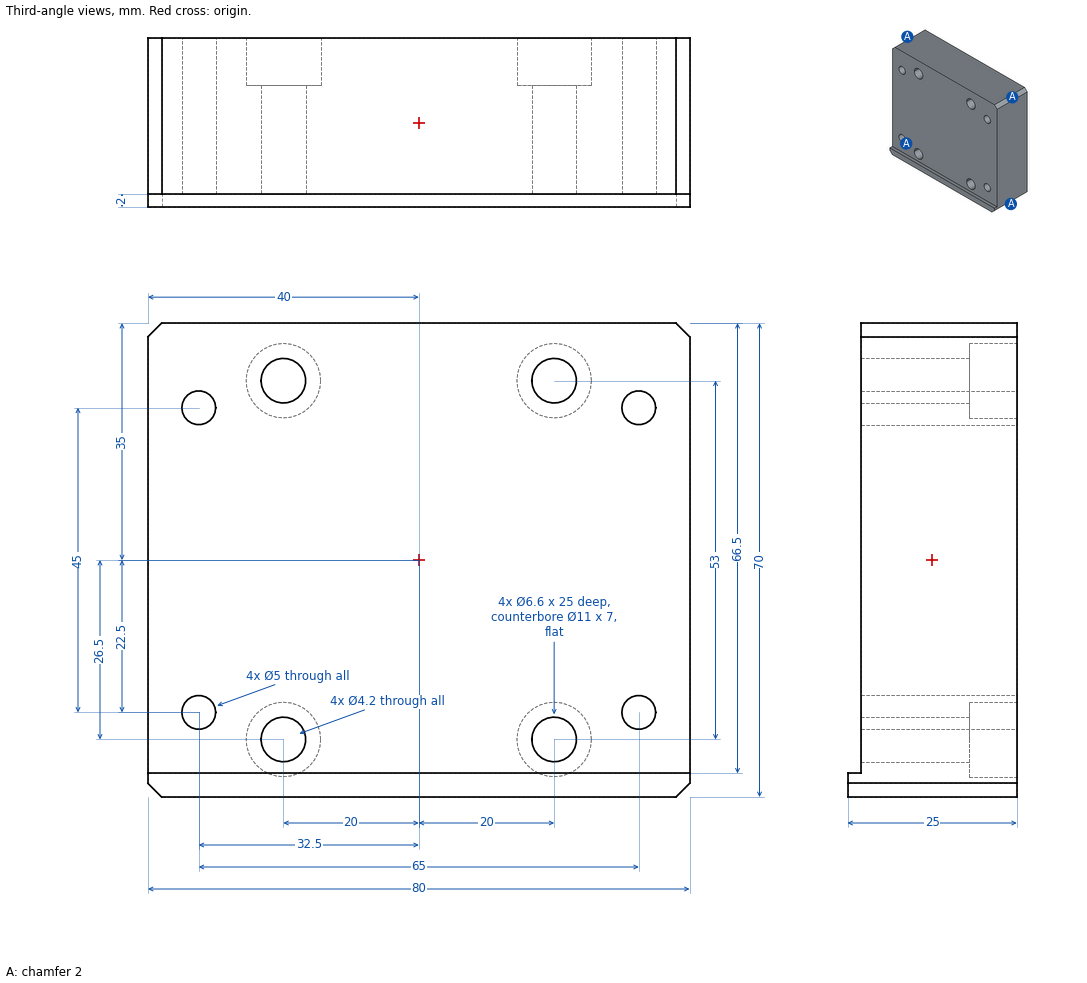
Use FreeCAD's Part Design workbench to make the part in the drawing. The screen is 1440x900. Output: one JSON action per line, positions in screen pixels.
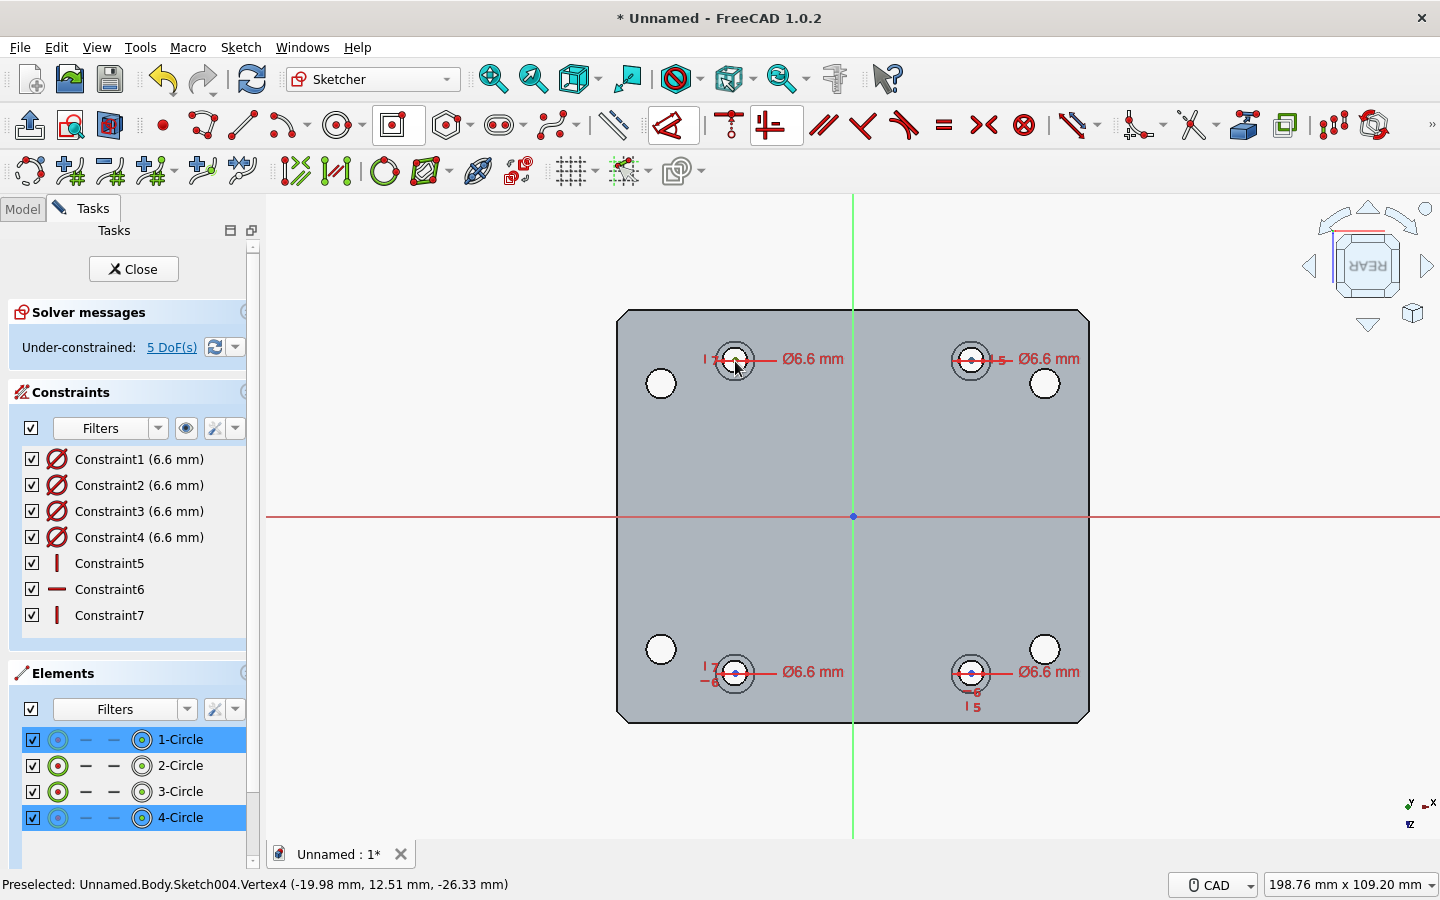
{"action": "key", "text": "h"}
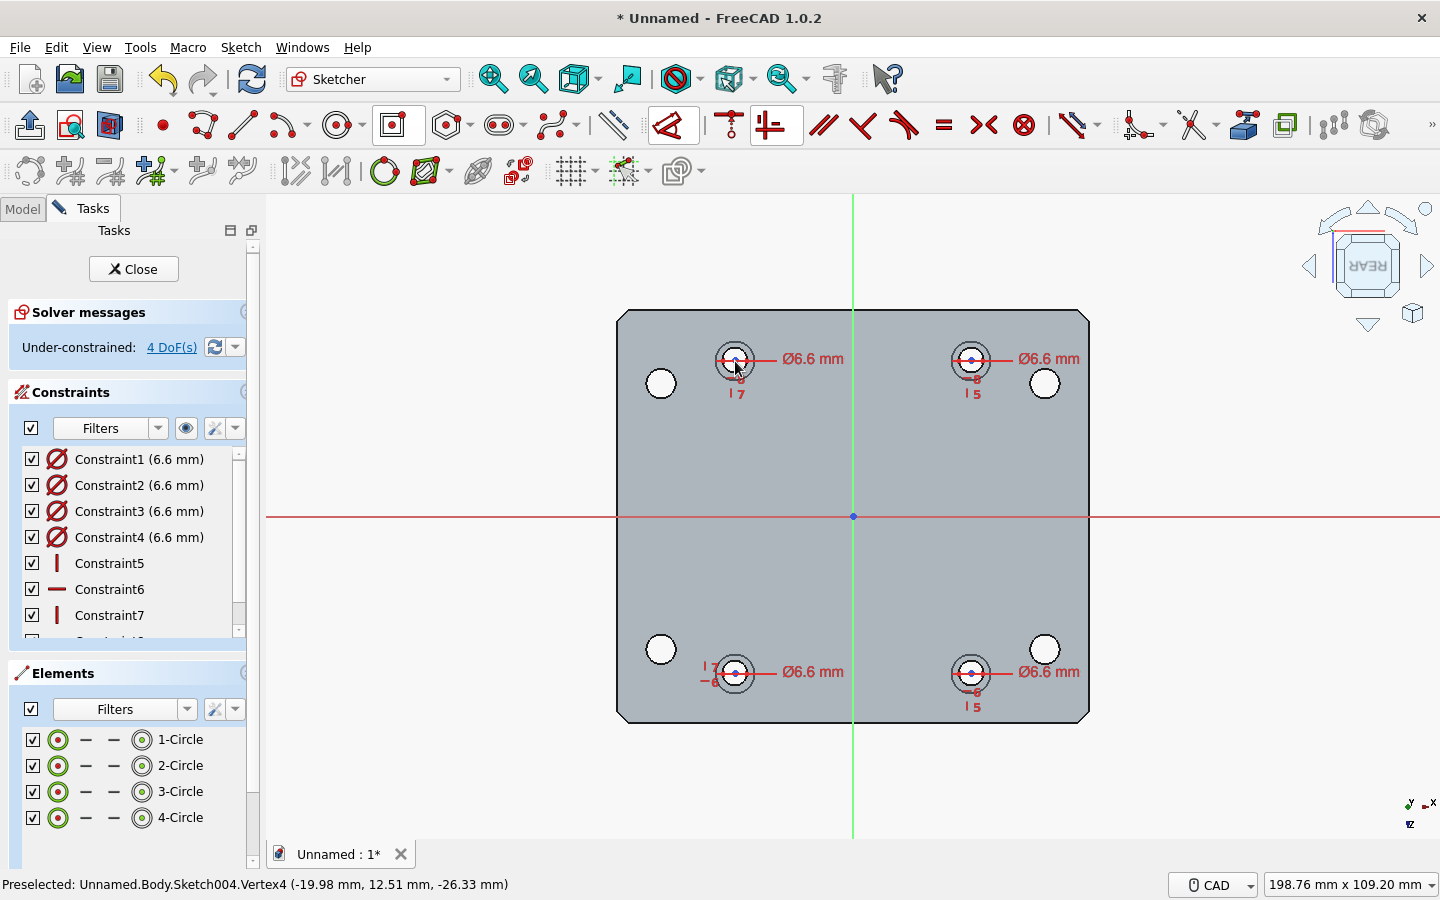
{"action": "left_click", "coordinate": [971, 361]}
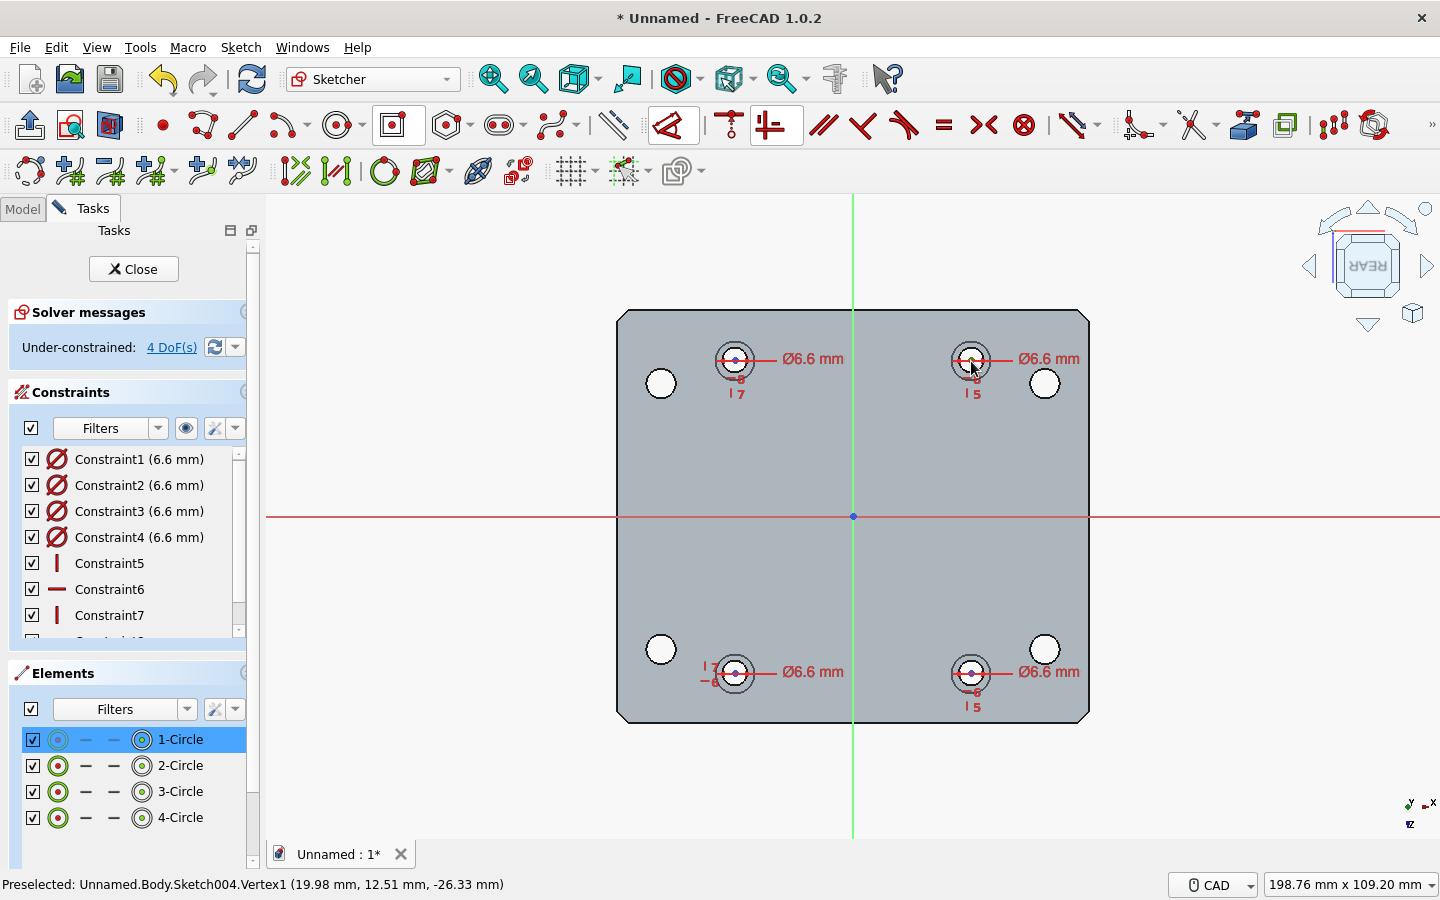
{"action": "left_click", "coordinate": [694, 126]}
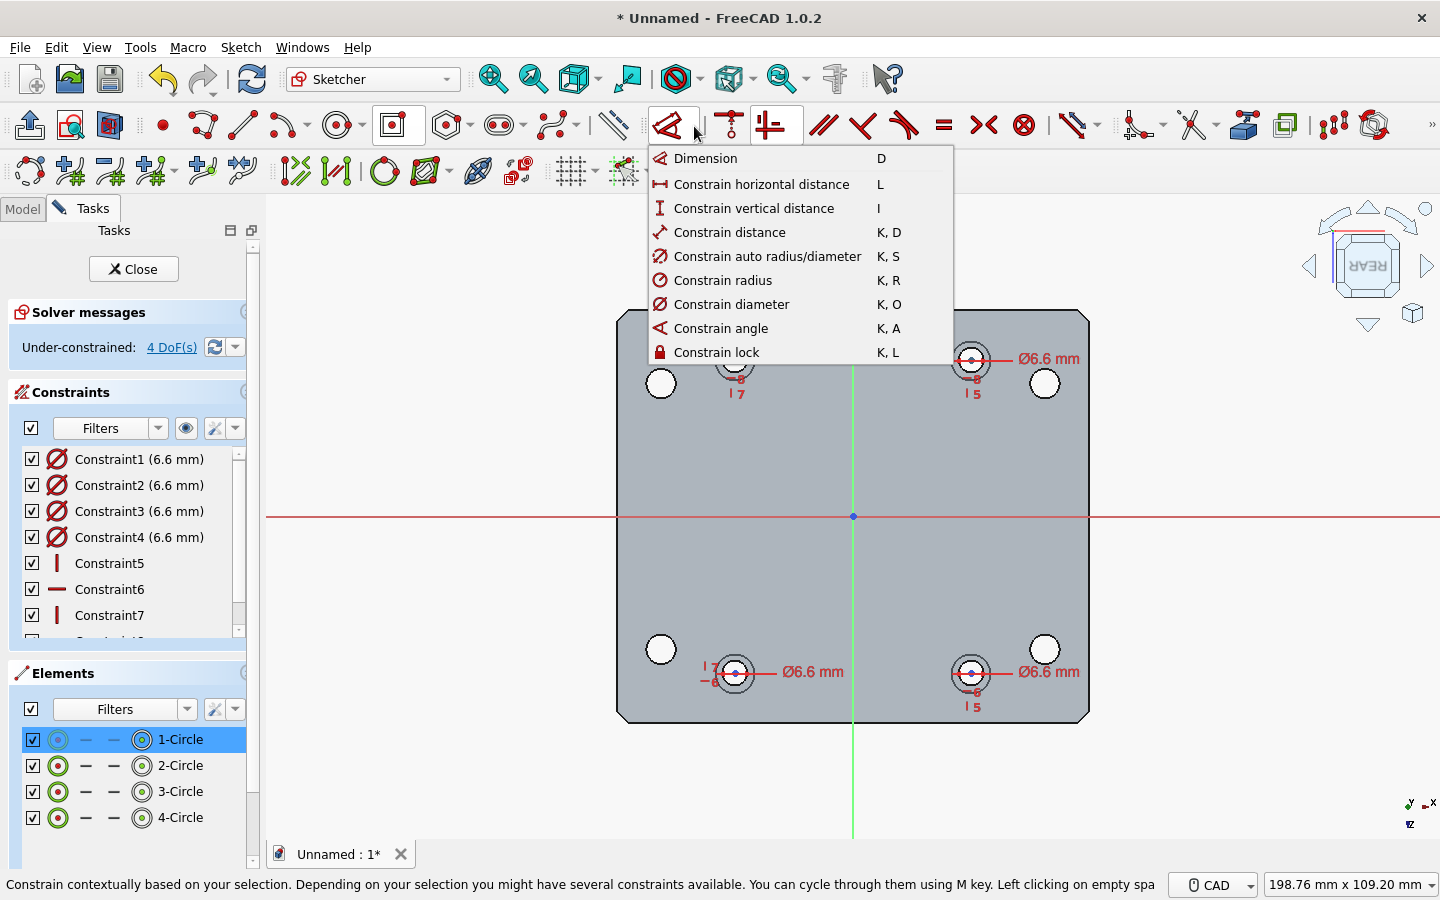
{"action": "left_click", "coordinate": [801, 184]}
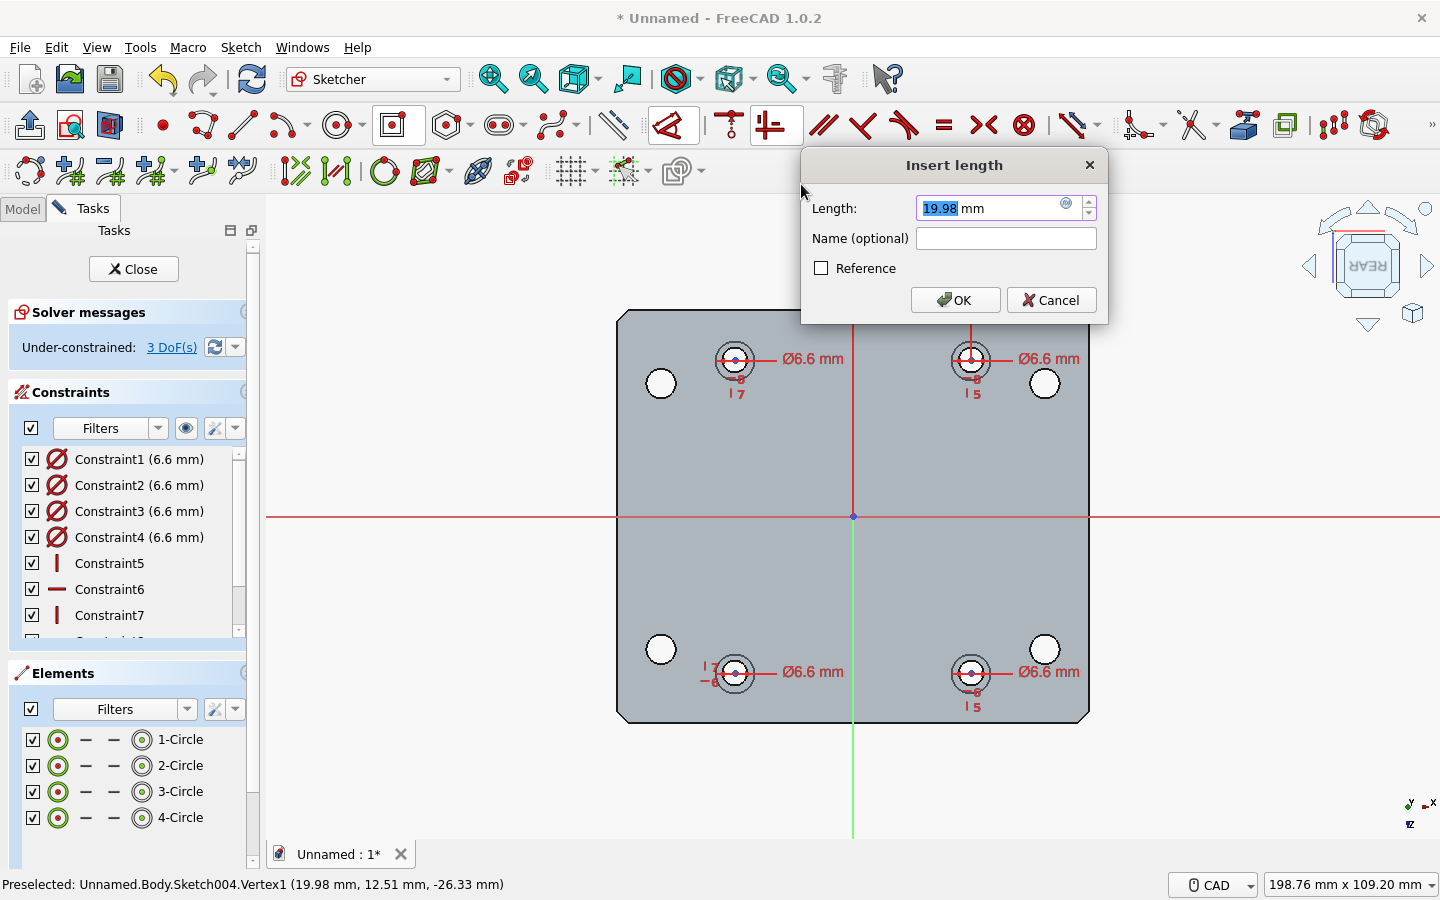
{"action": "type", "text": "20"}
{"action": "key", "text": "Return"}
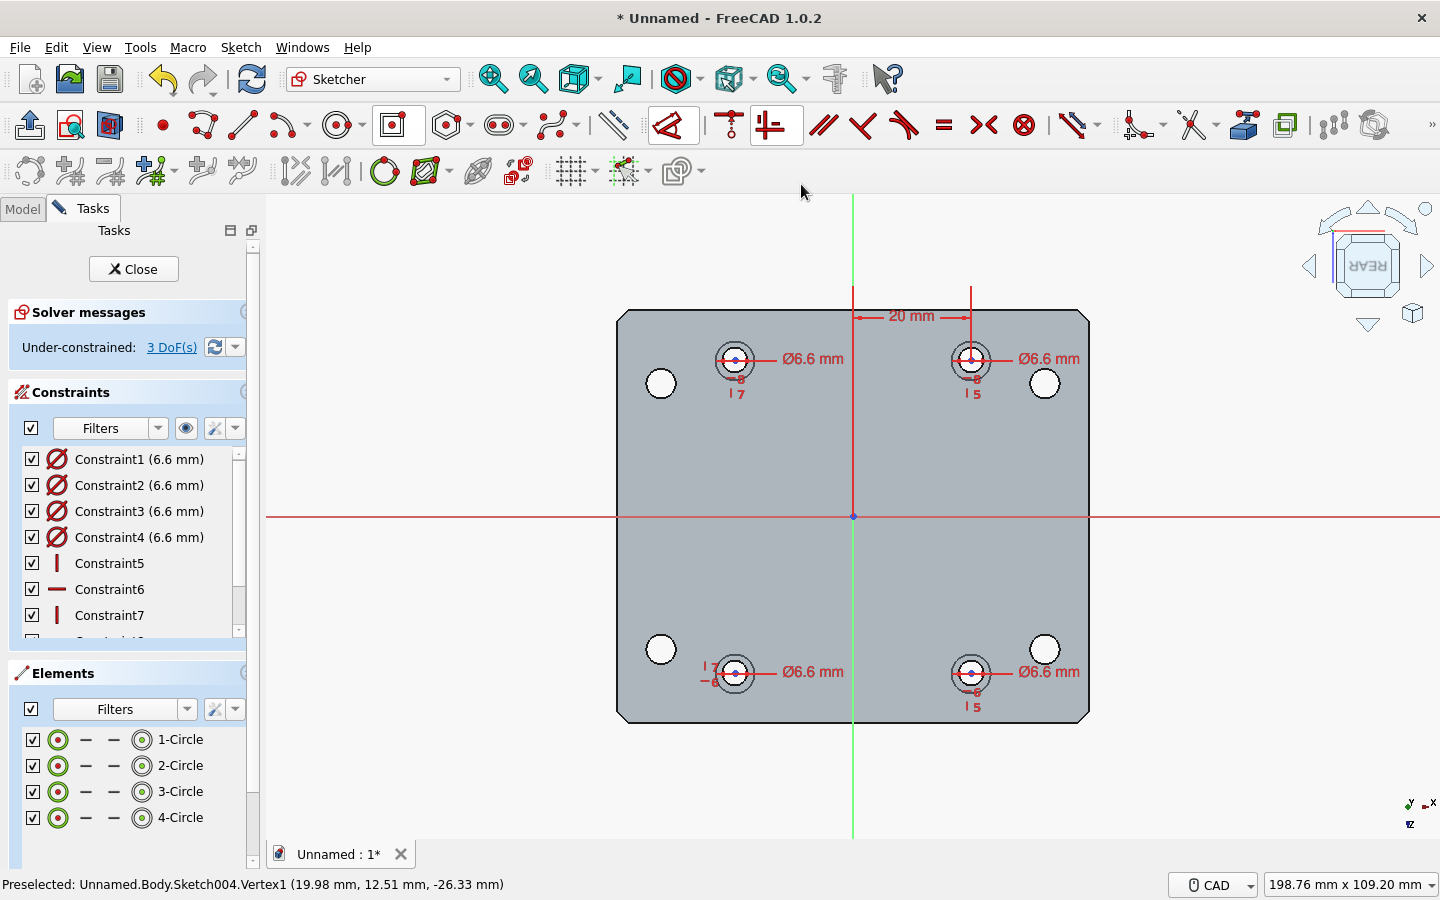
{"action": "left_click", "coordinate": [735, 674]}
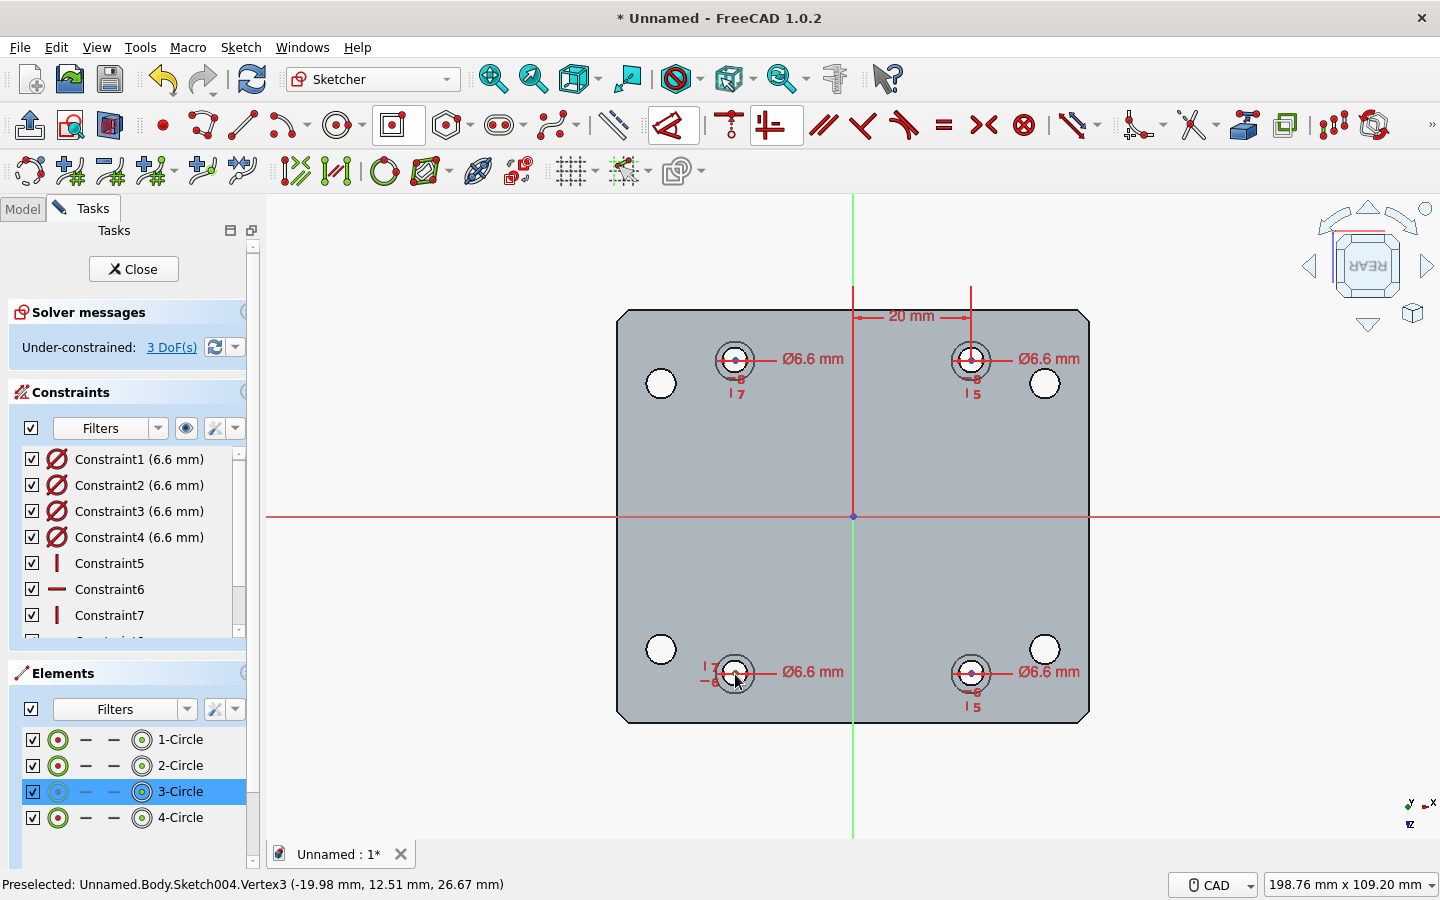
{"action": "left_click", "coordinate": [694, 126]}